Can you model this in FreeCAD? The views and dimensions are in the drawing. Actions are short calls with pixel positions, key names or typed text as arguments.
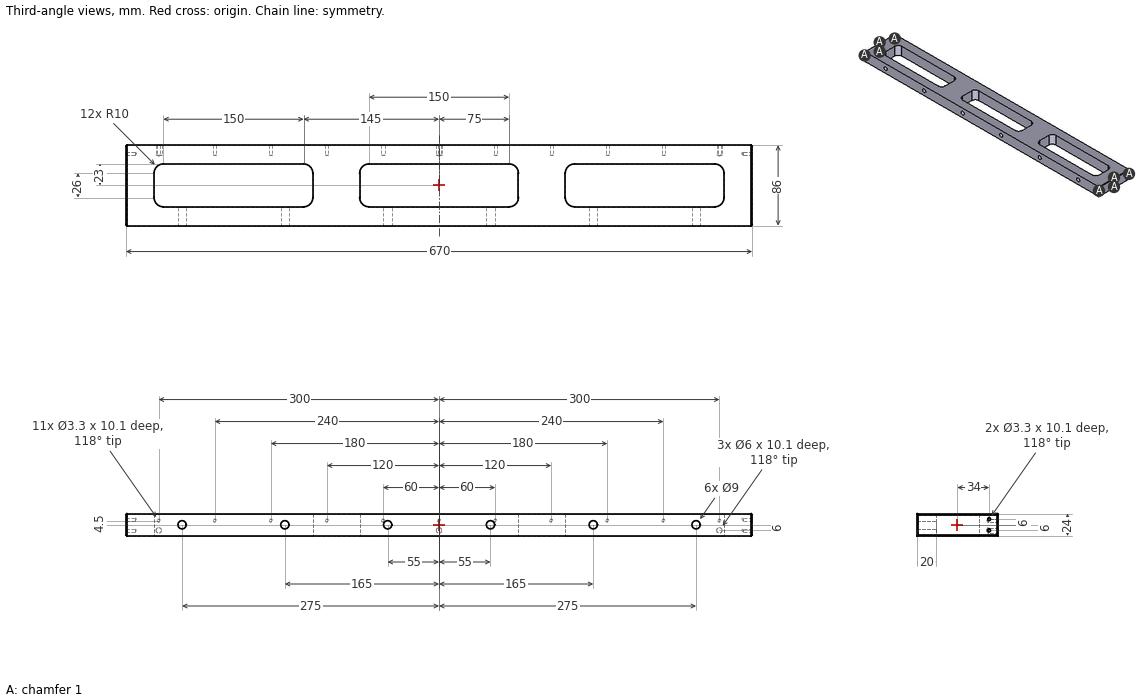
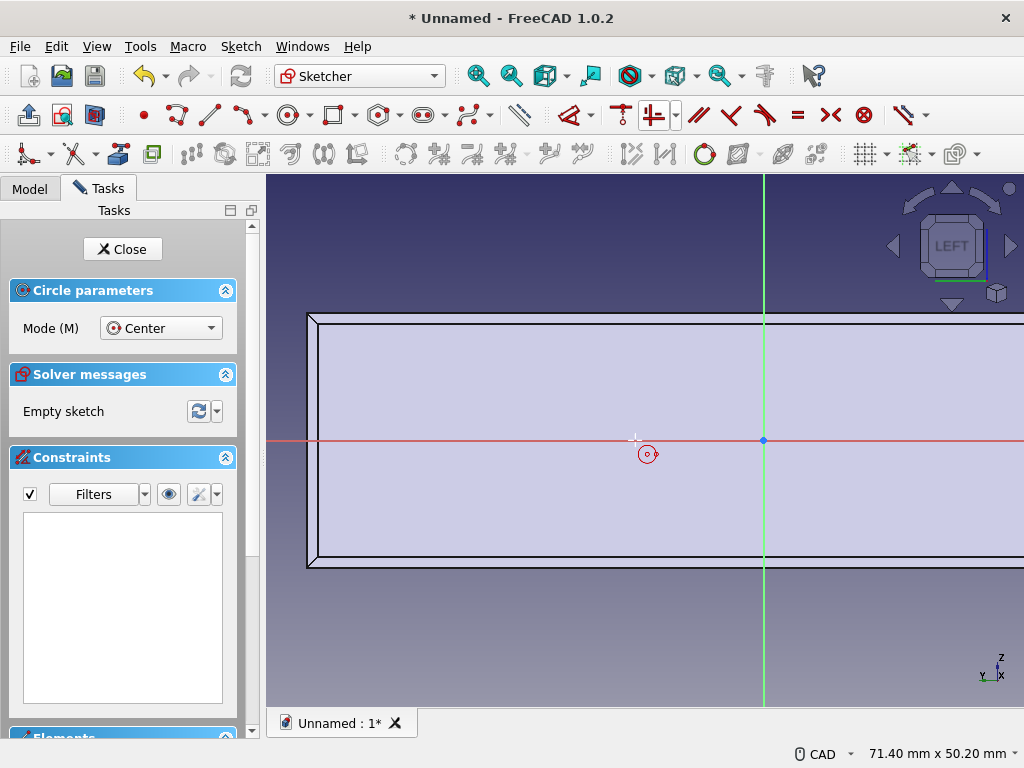
scroll(403, 377, up, 2)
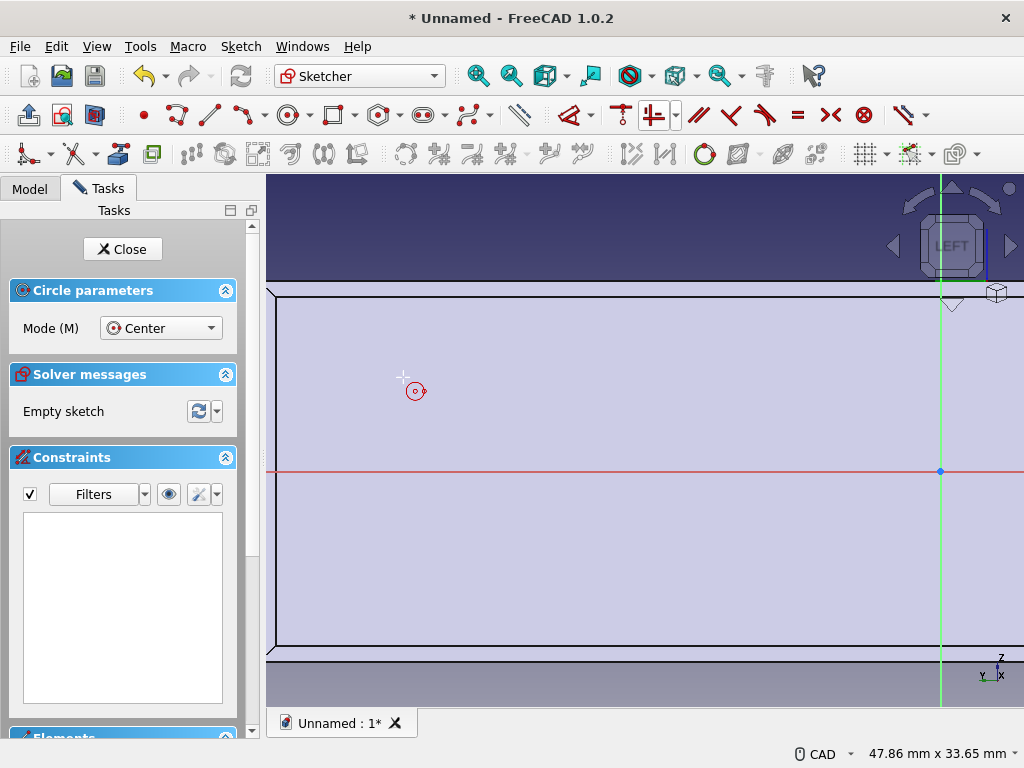
click(402, 377)
move(421, 358)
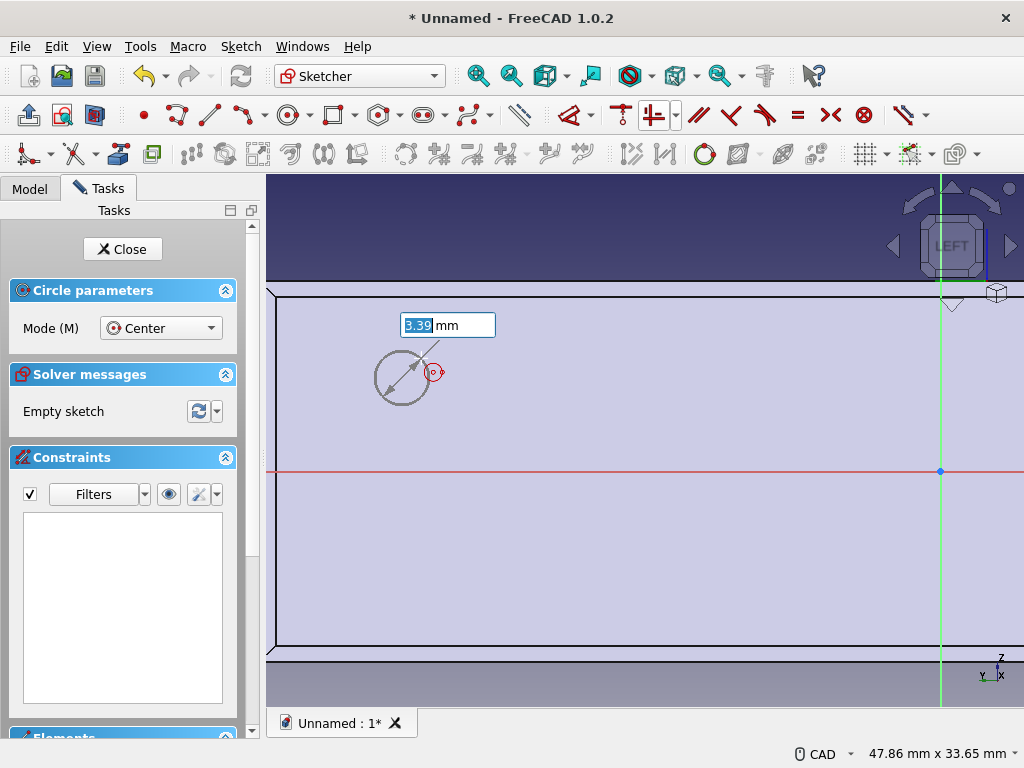
text(3.3)
key(Return)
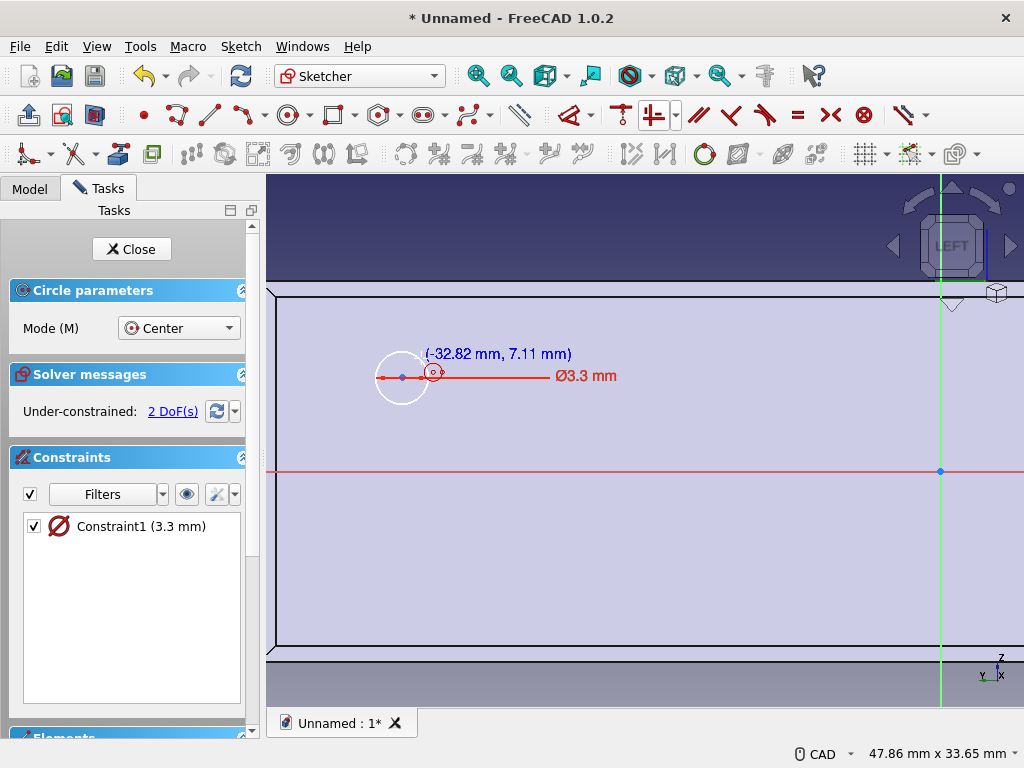
click(402, 567)
move(421, 548)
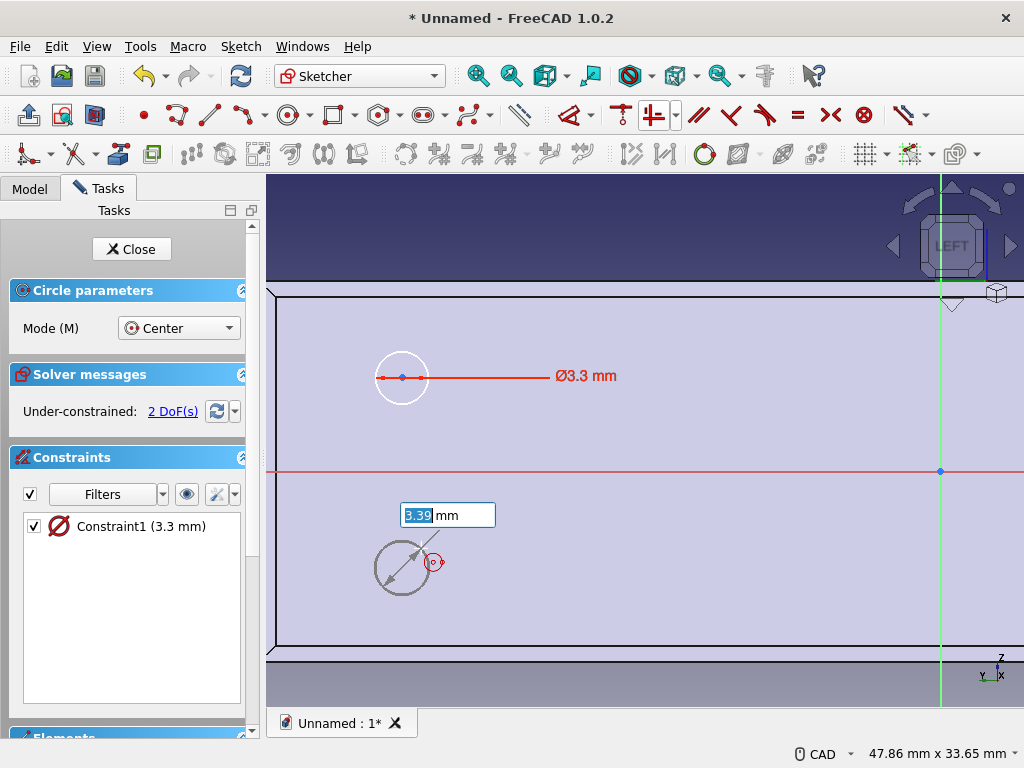
text(3.3)
key(Return)
key(Escape)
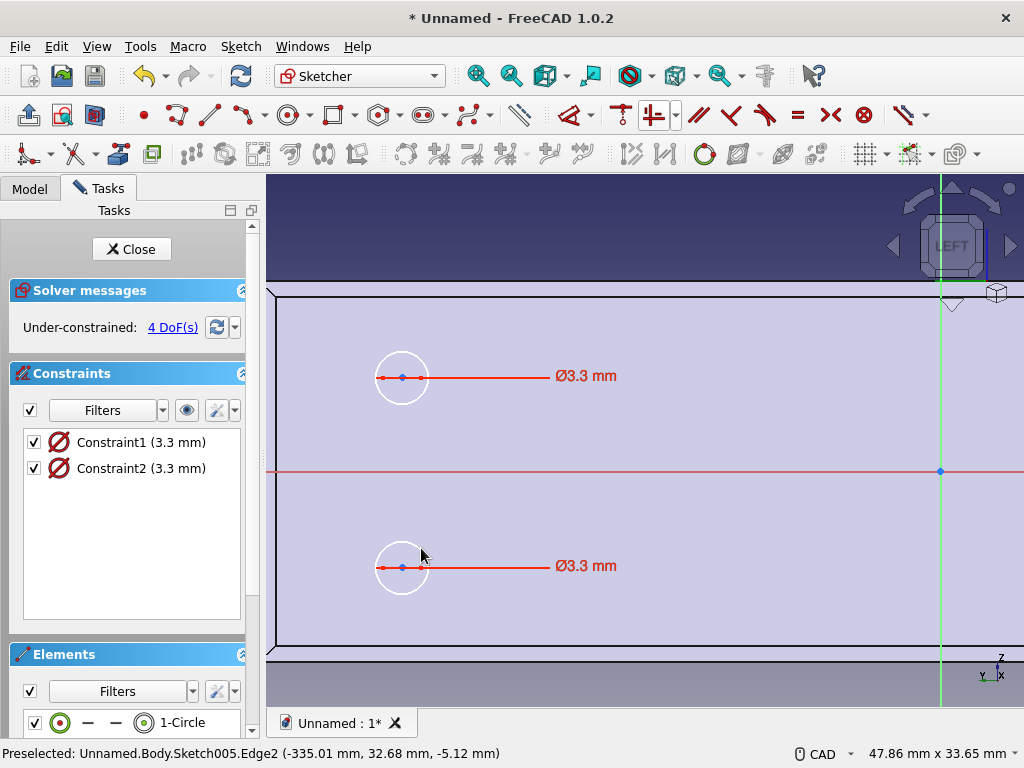
click(402, 378)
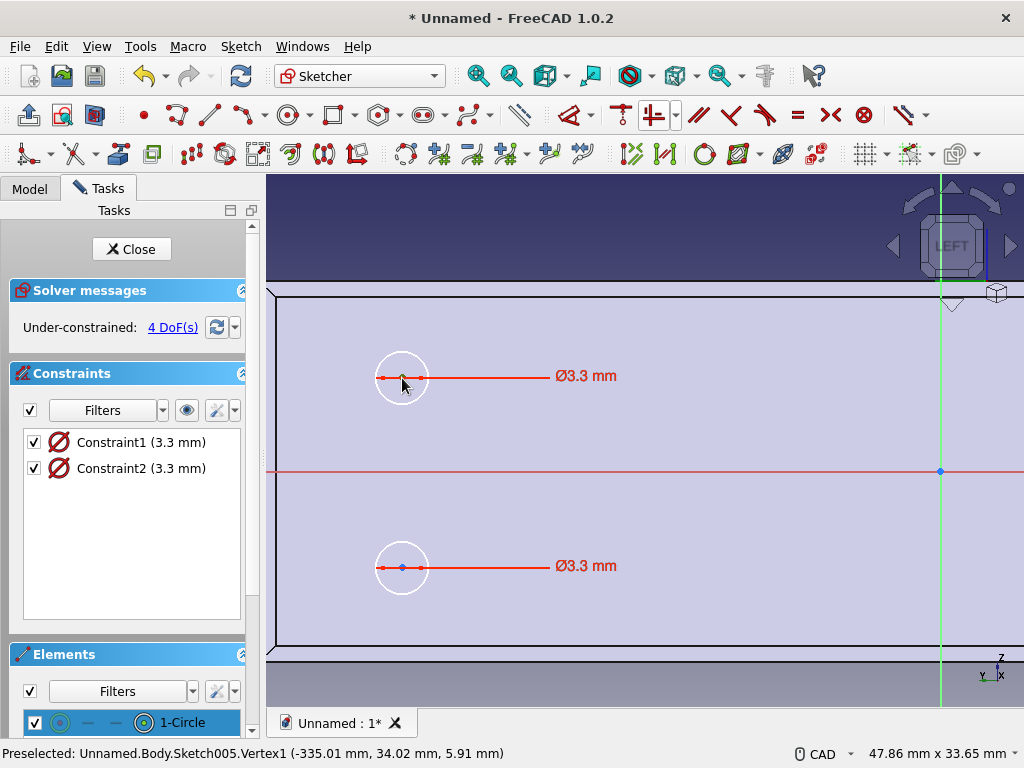
click(402, 568)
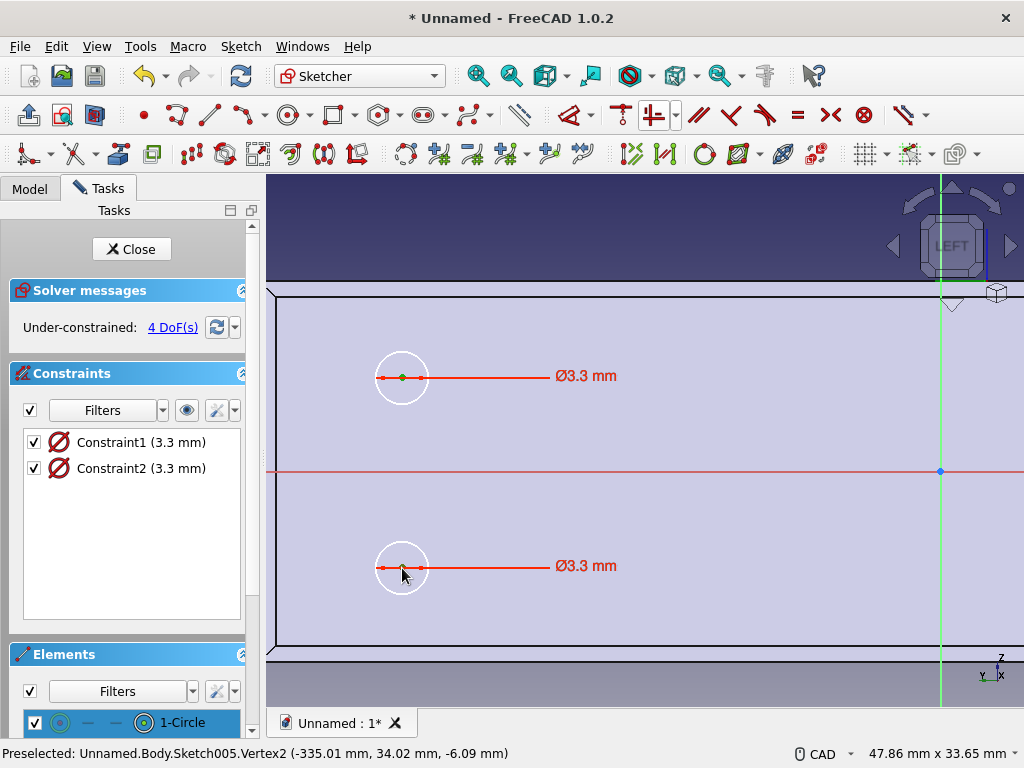
key(v)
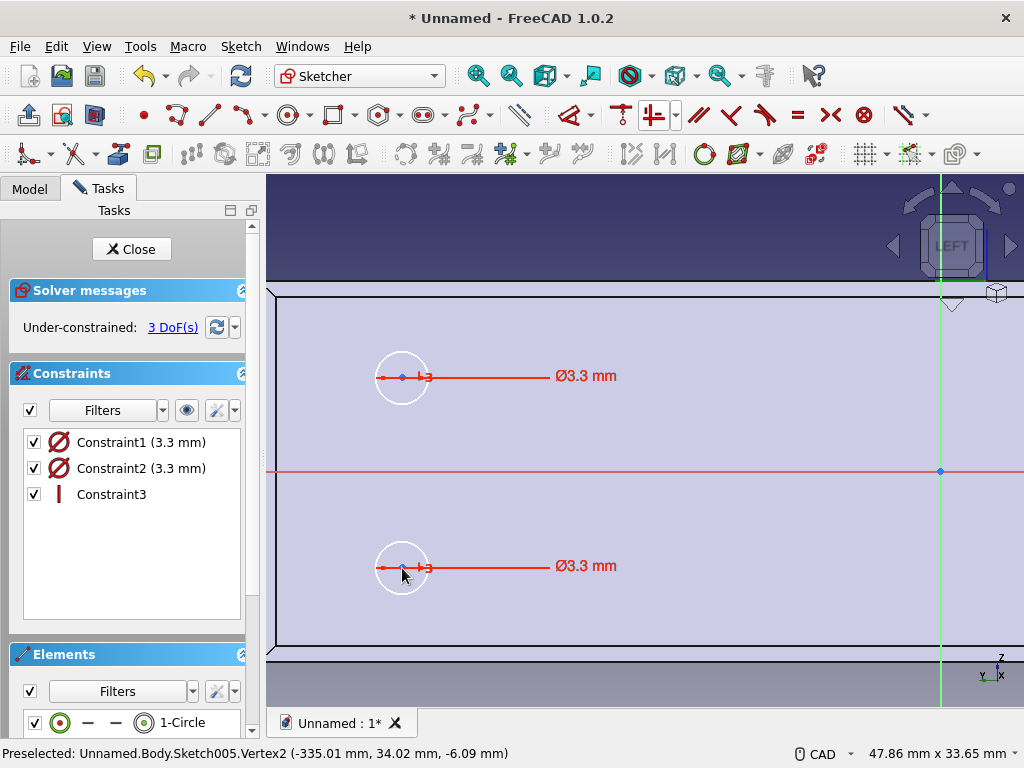
key(d)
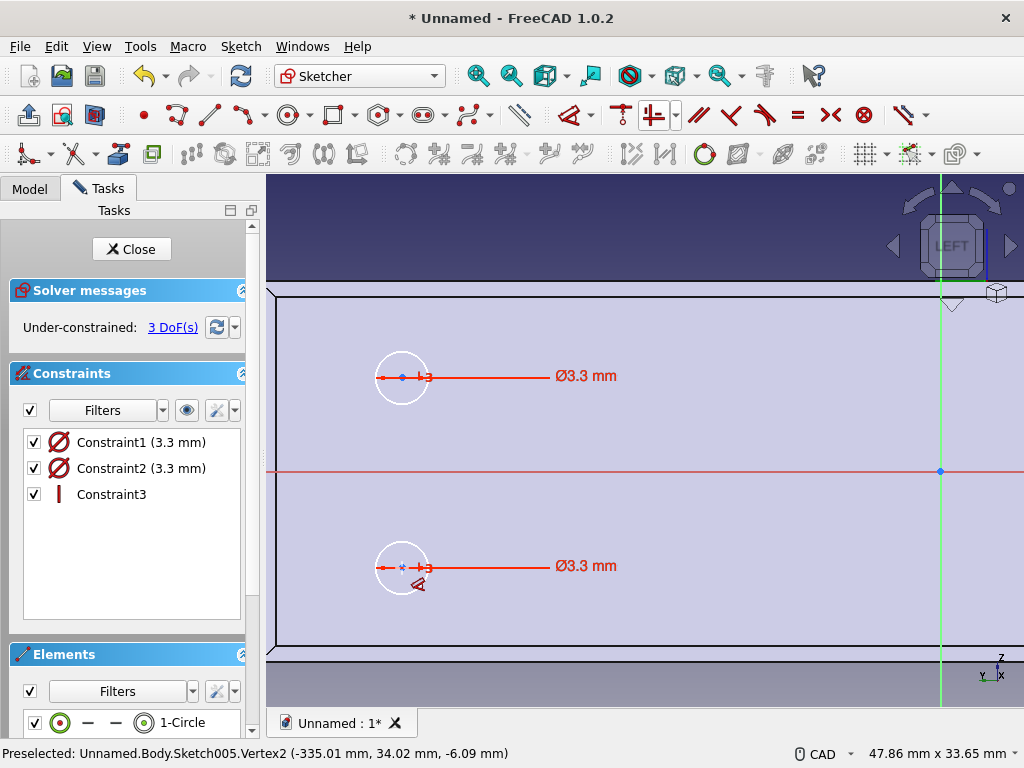
click(402, 378)
click(368, 425)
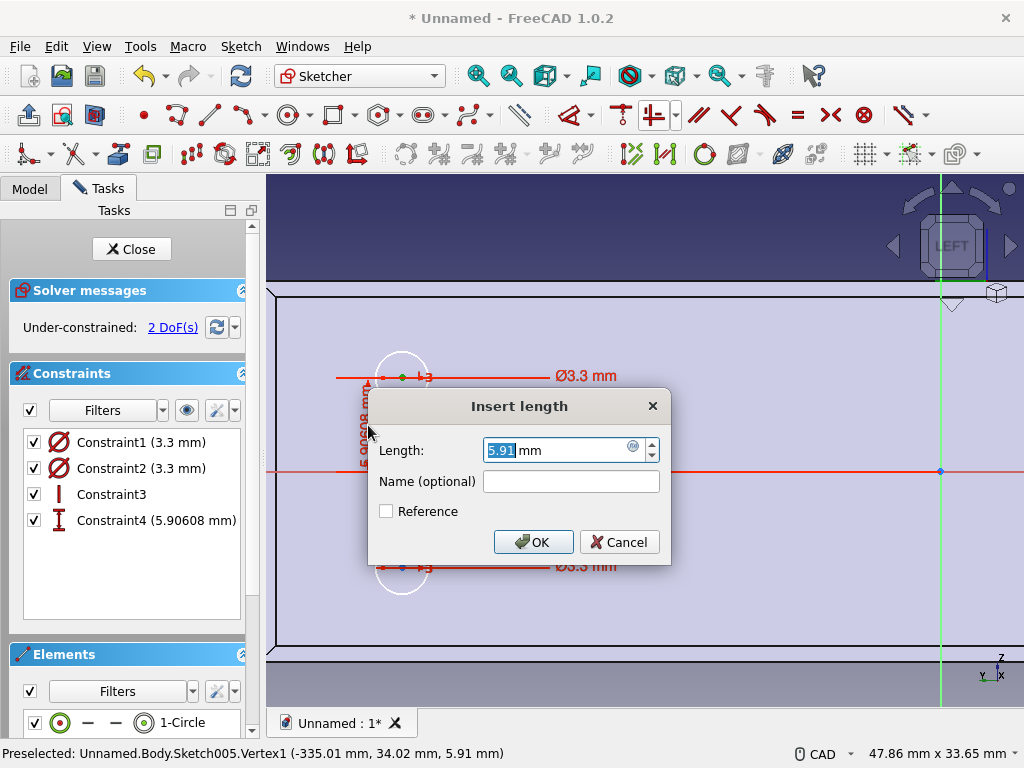
text(6)
key(Return)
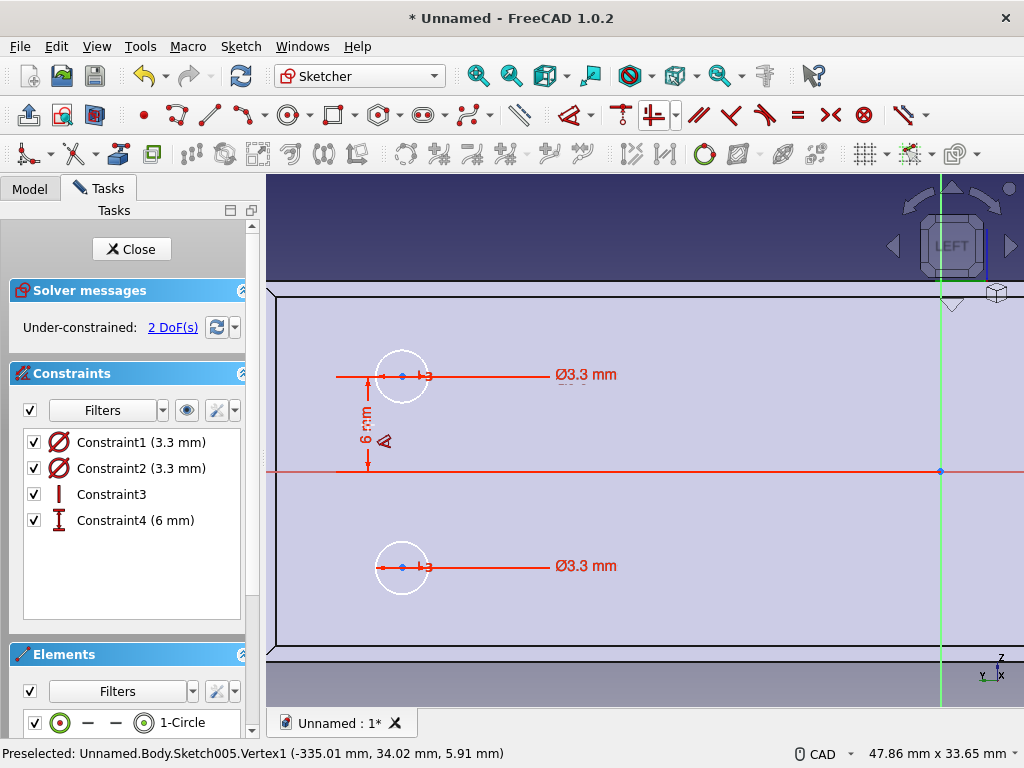
click(402, 568)
click(368, 520)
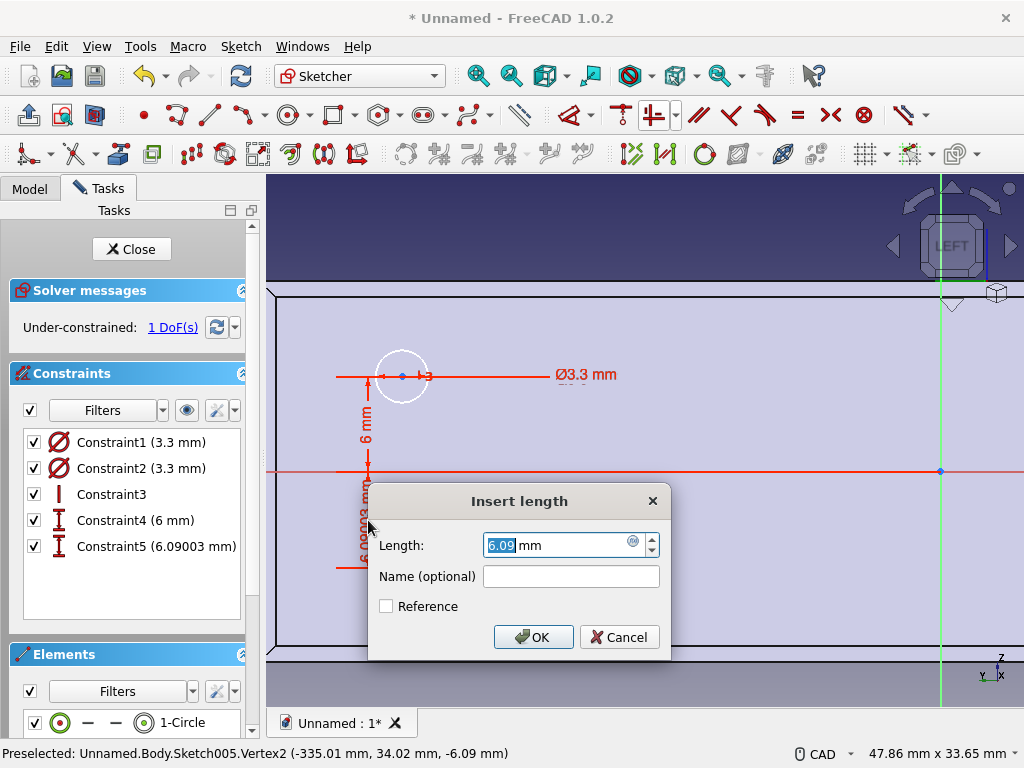
text(6)
key(Return)